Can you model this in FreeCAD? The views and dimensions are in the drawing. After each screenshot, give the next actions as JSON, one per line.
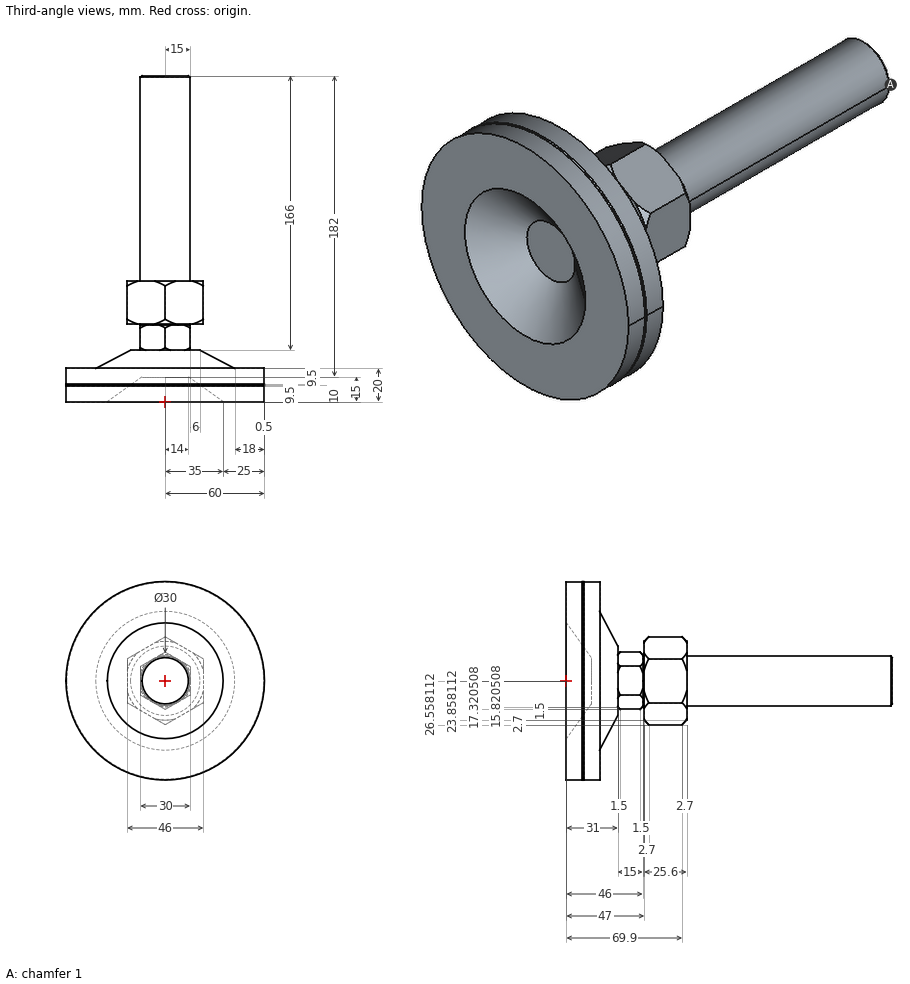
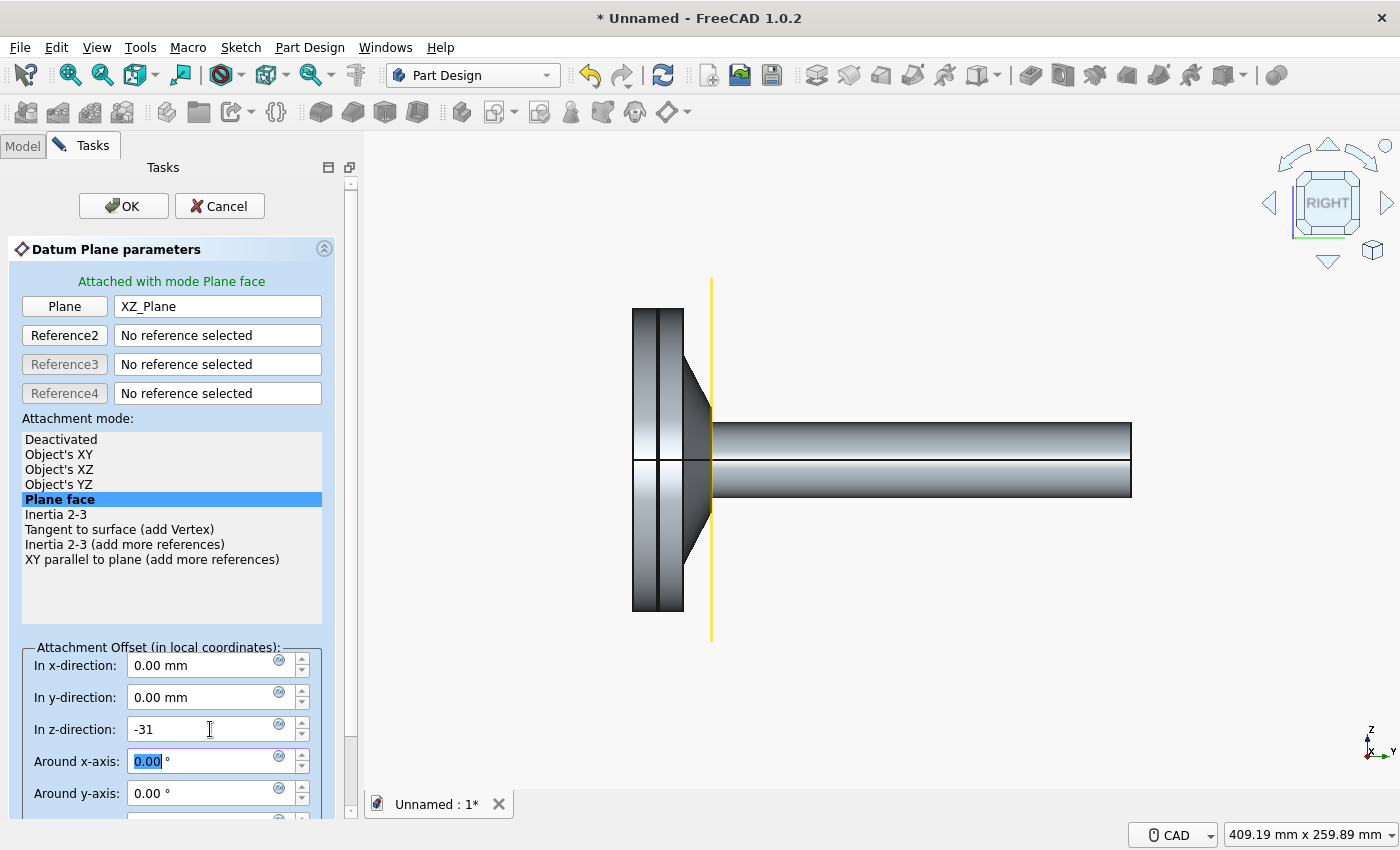
{"action": "left_click", "coordinate": [124, 206]}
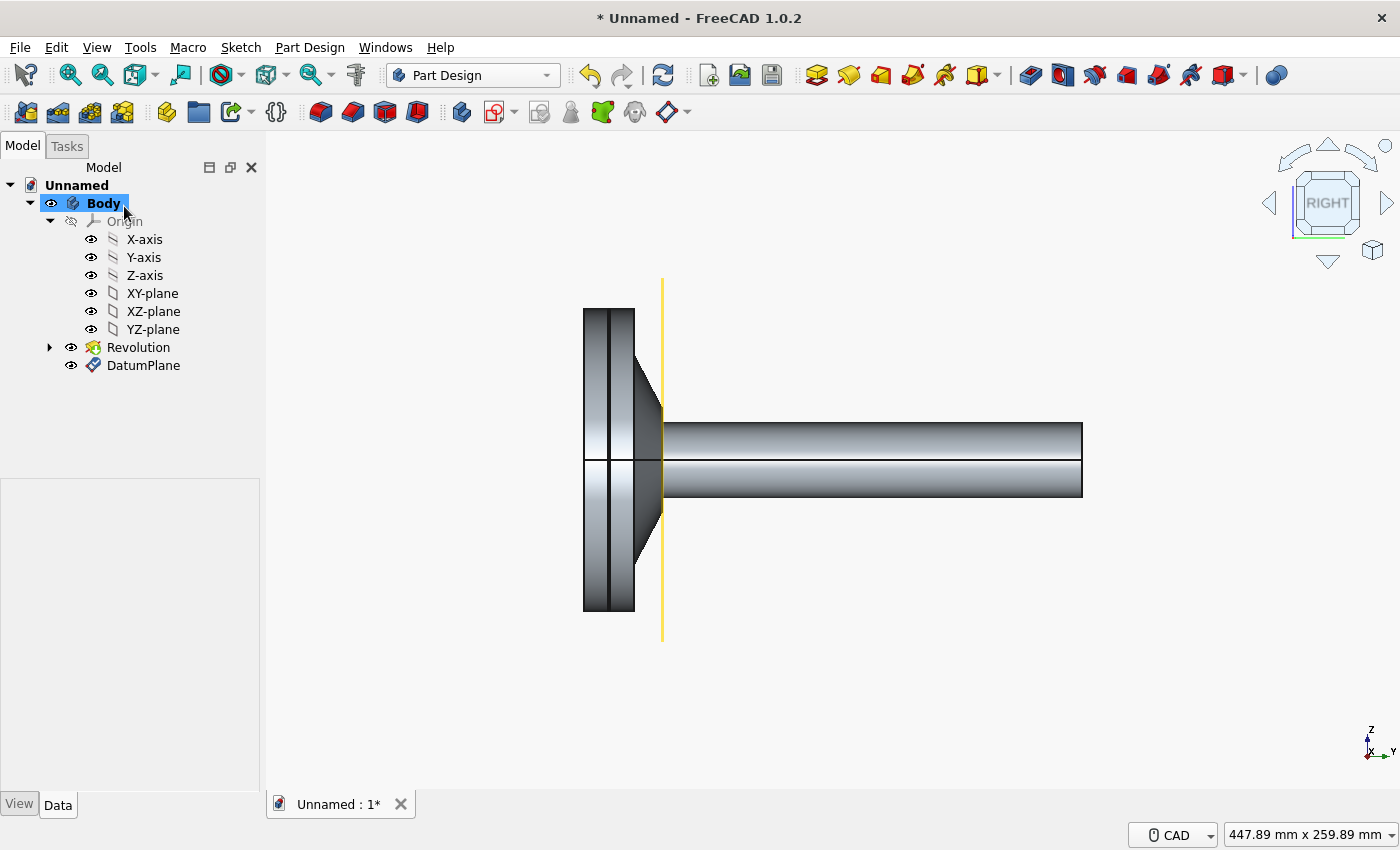
{"action": "left_click", "coordinate": [116, 365]}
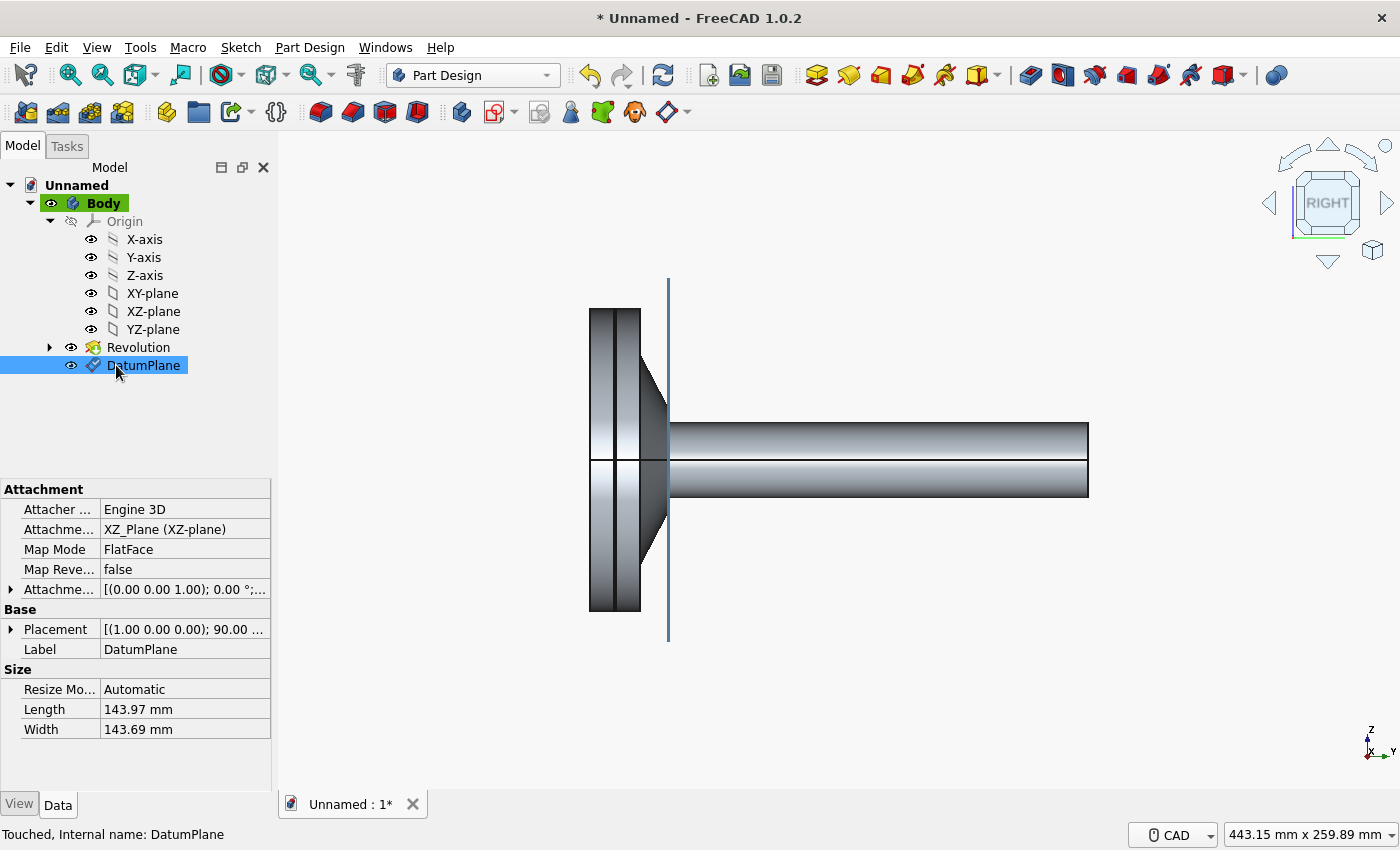
{"action": "left_click", "coordinate": [494, 112]}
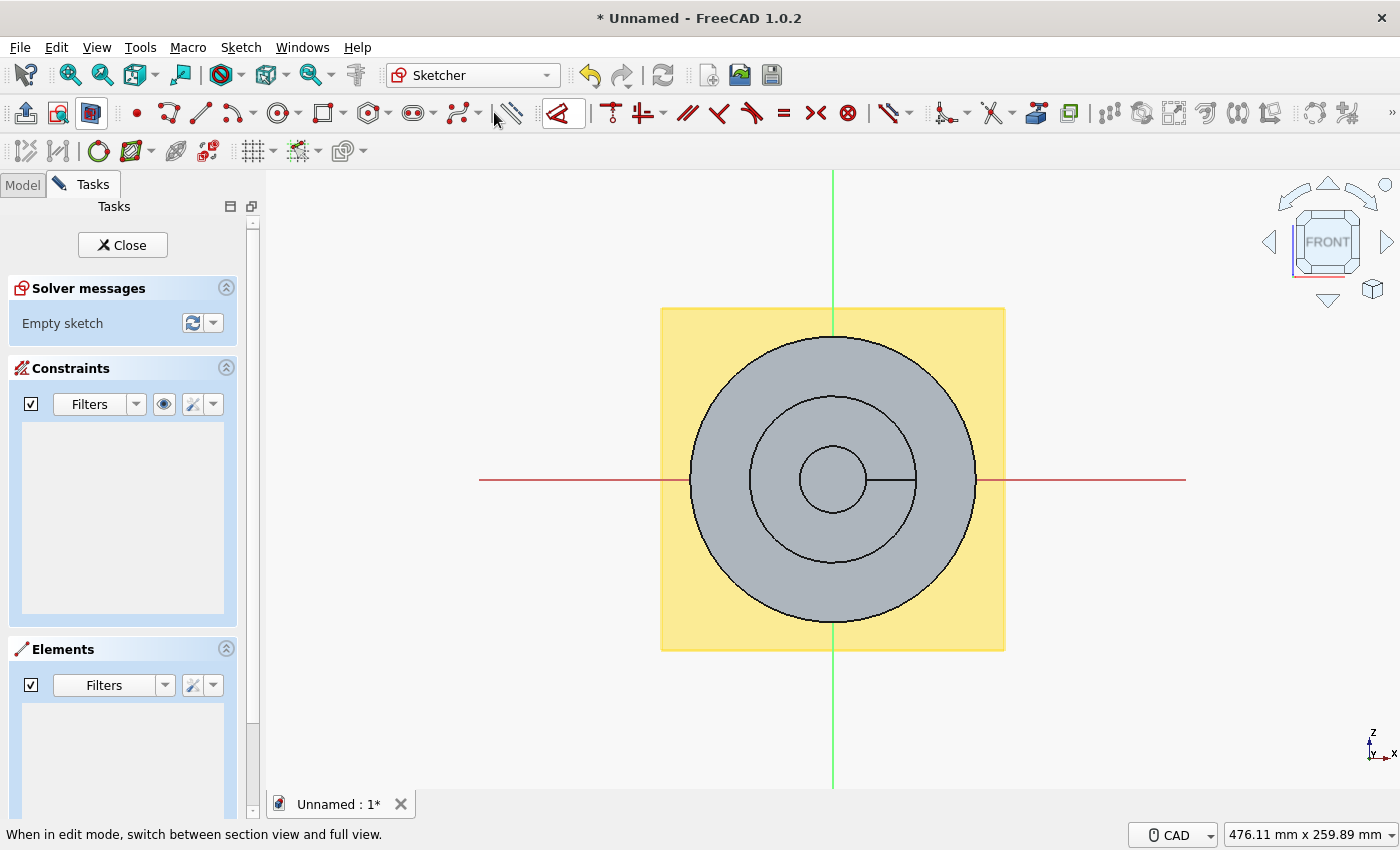
{"action": "left_click", "coordinate": [92, 114]}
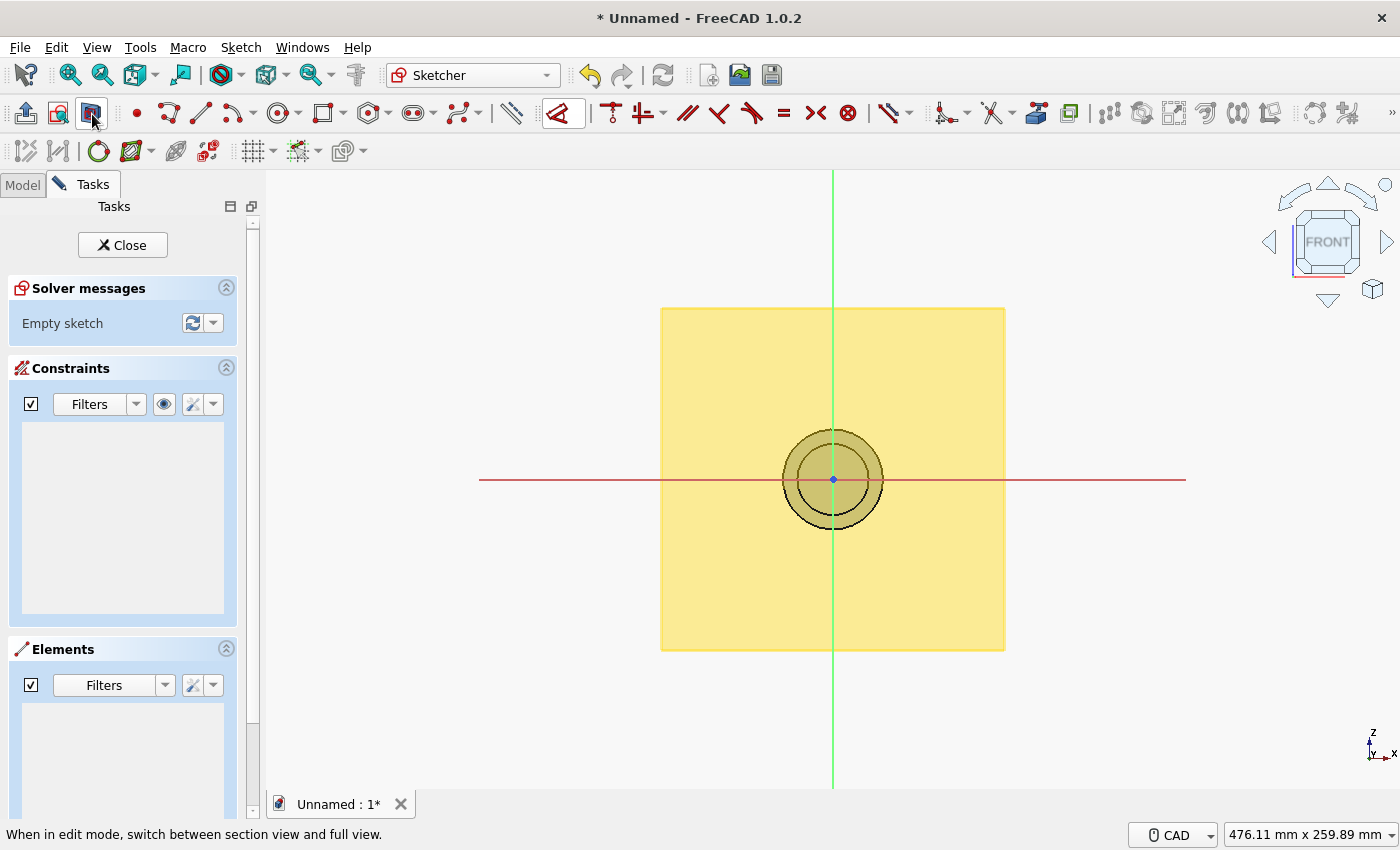
{"action": "scroll", "coordinate": [850, 479], "scroll_direction": "up", "scroll_amount": 8}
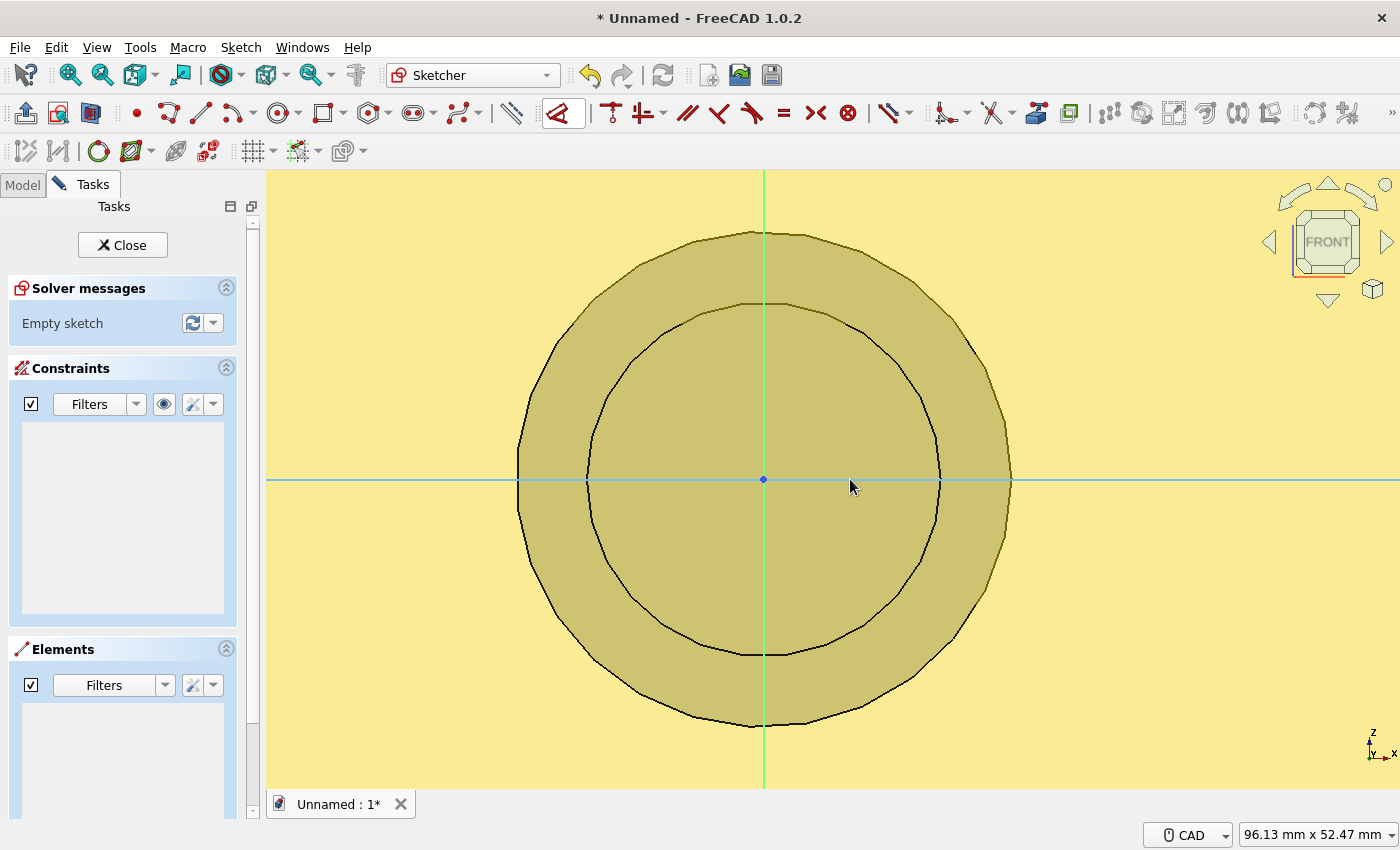
{"action": "left_click", "coordinate": [368, 114]}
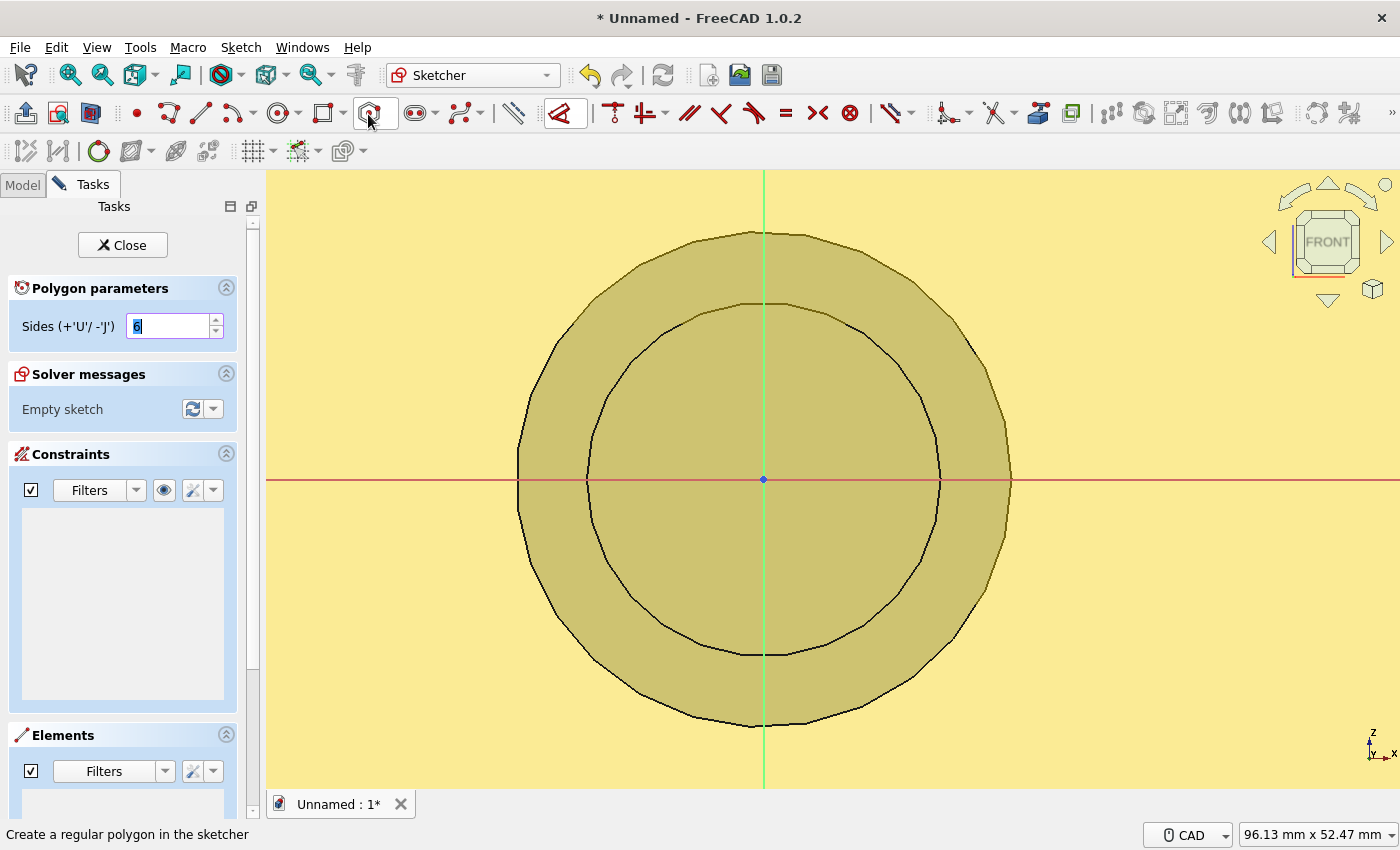
{"action": "left_click", "coordinate": [764, 479]}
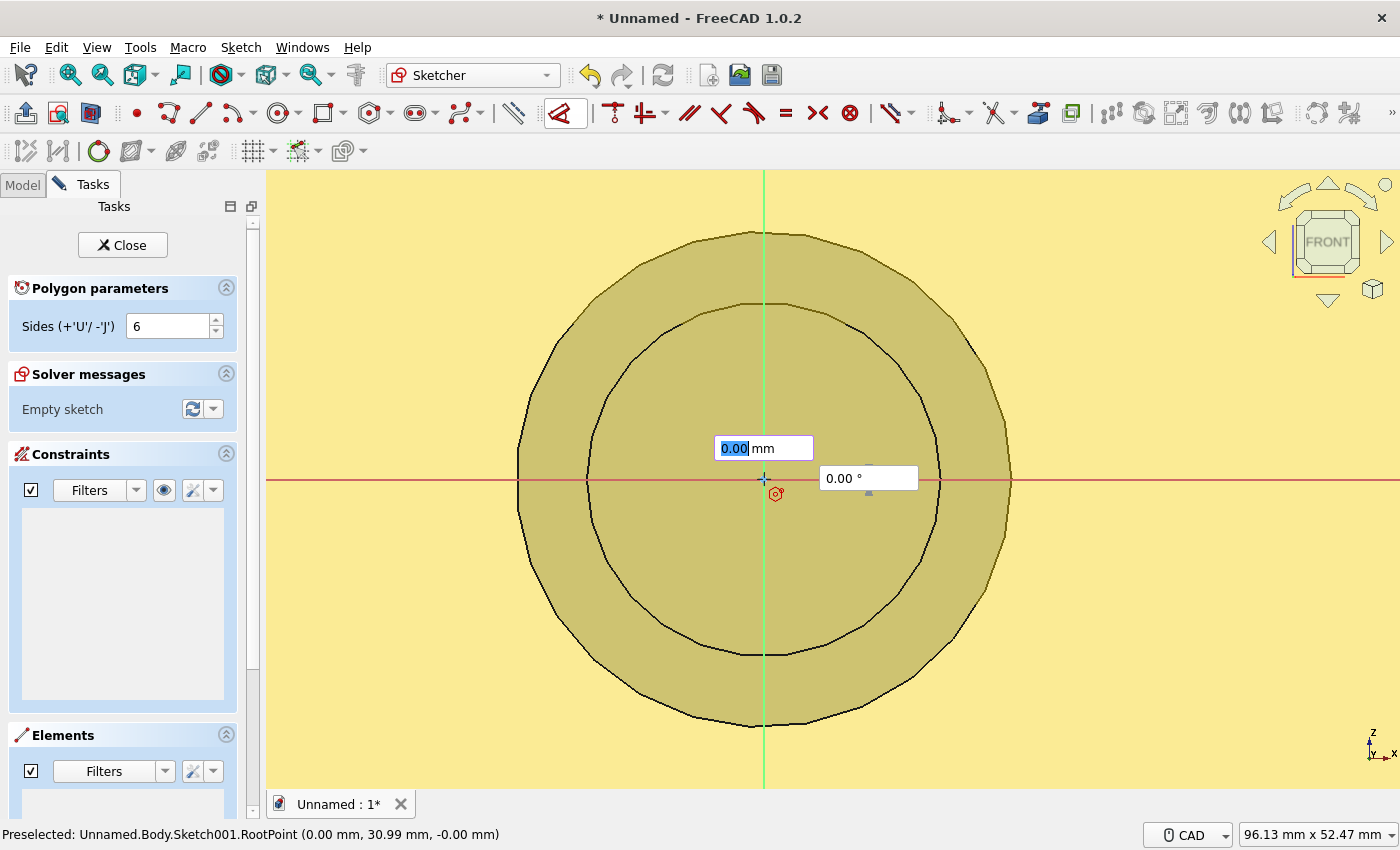
{"action": "left_click", "coordinate": [764, 684]}
{"action": "right_click", "coordinate": [764, 684]}